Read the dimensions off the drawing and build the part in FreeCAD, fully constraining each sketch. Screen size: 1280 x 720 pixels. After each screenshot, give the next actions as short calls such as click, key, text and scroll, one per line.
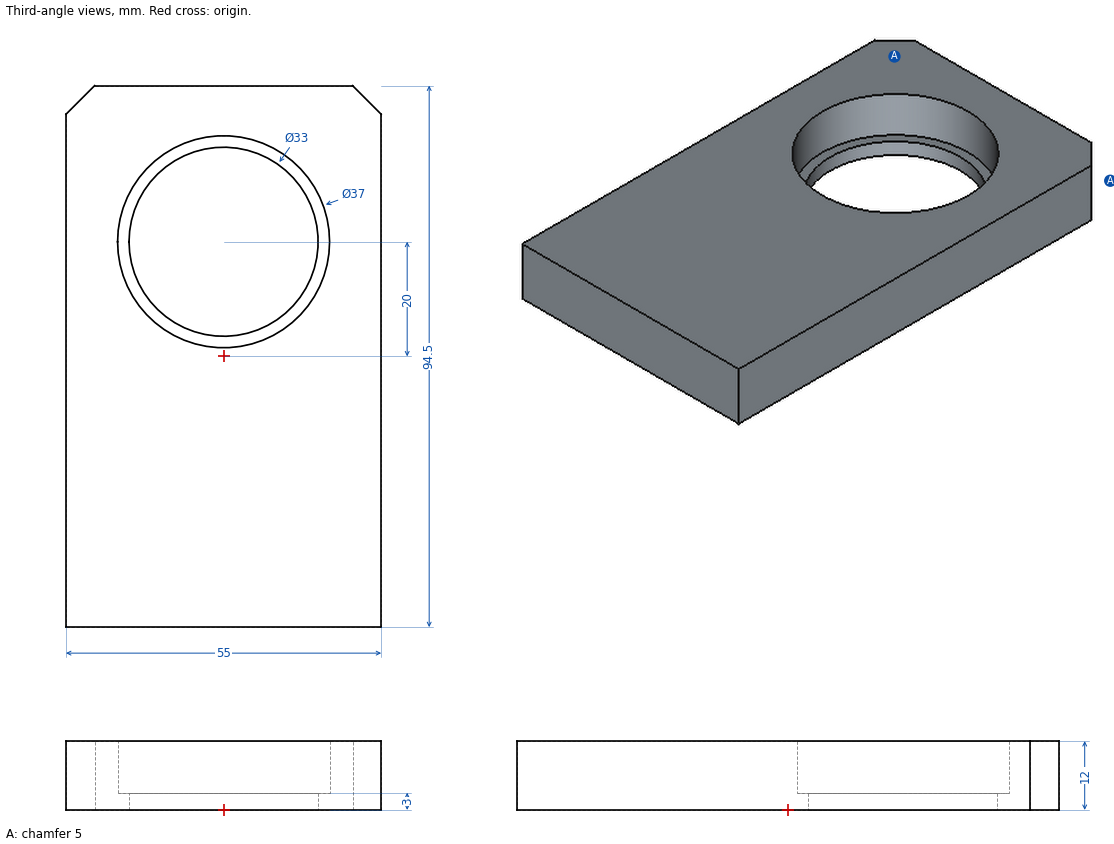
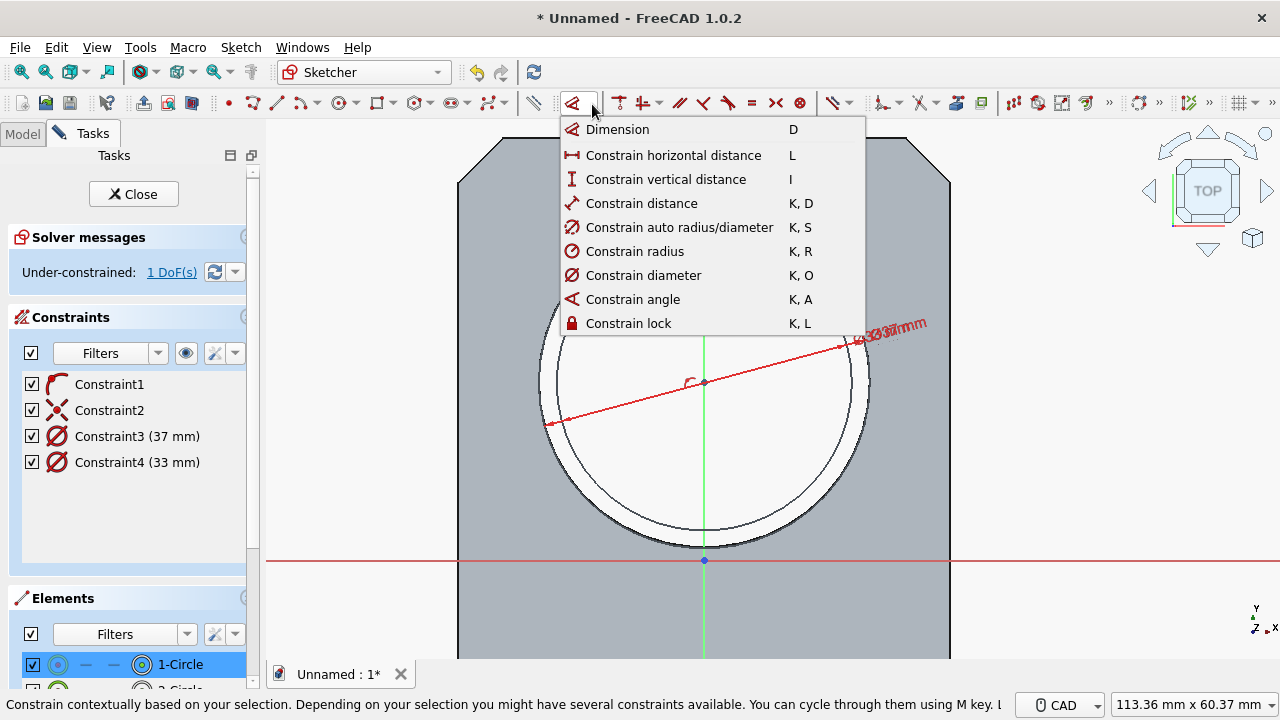
click(713, 179)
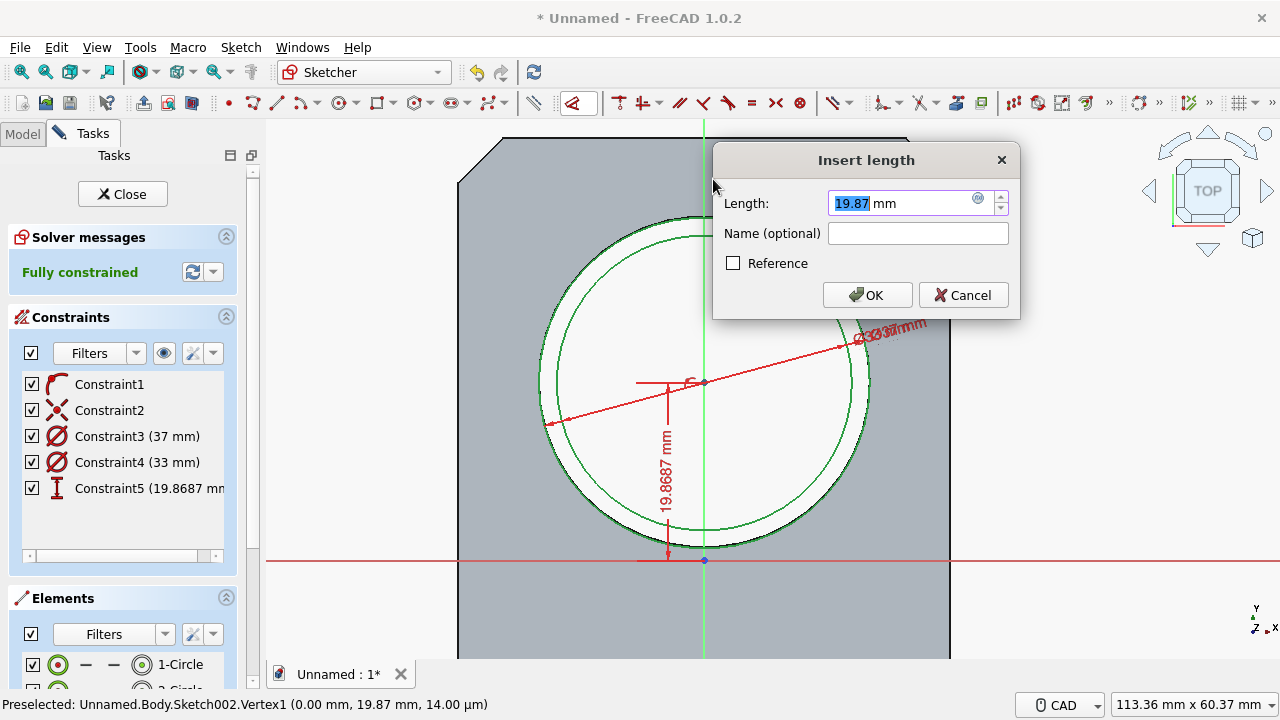
text(20)
key(Return)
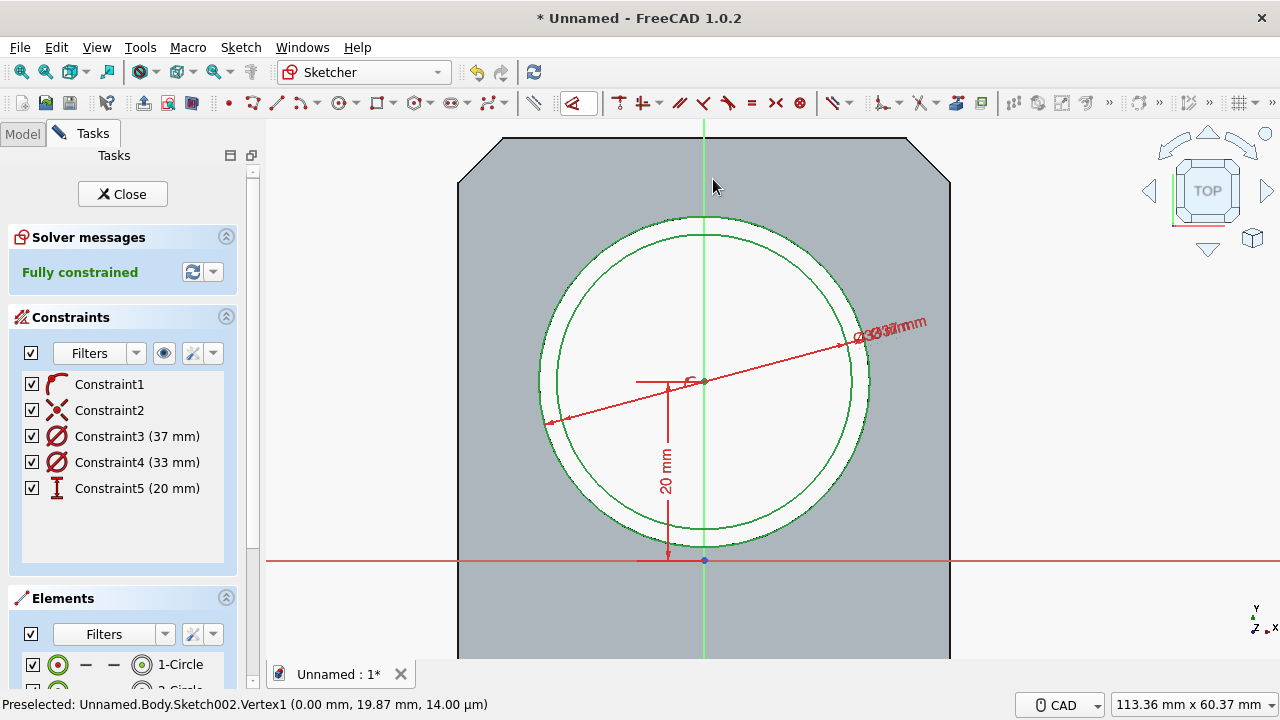
click(123, 194)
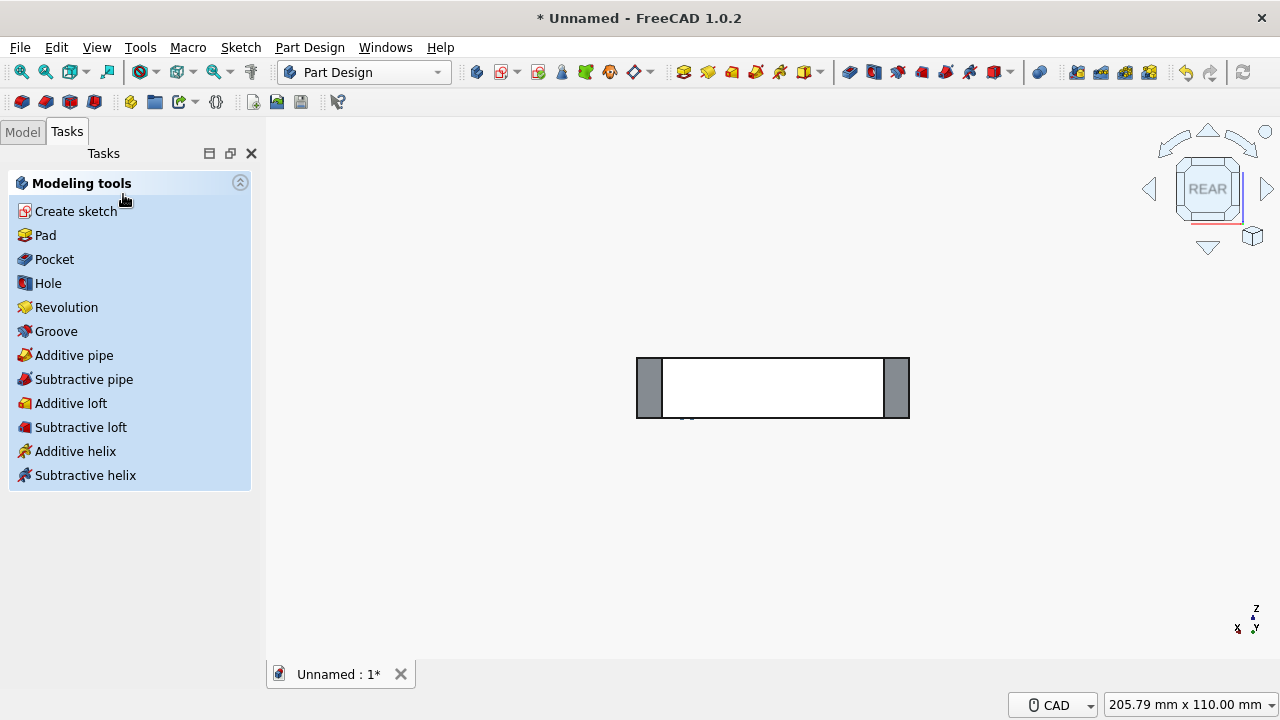
click(684, 72)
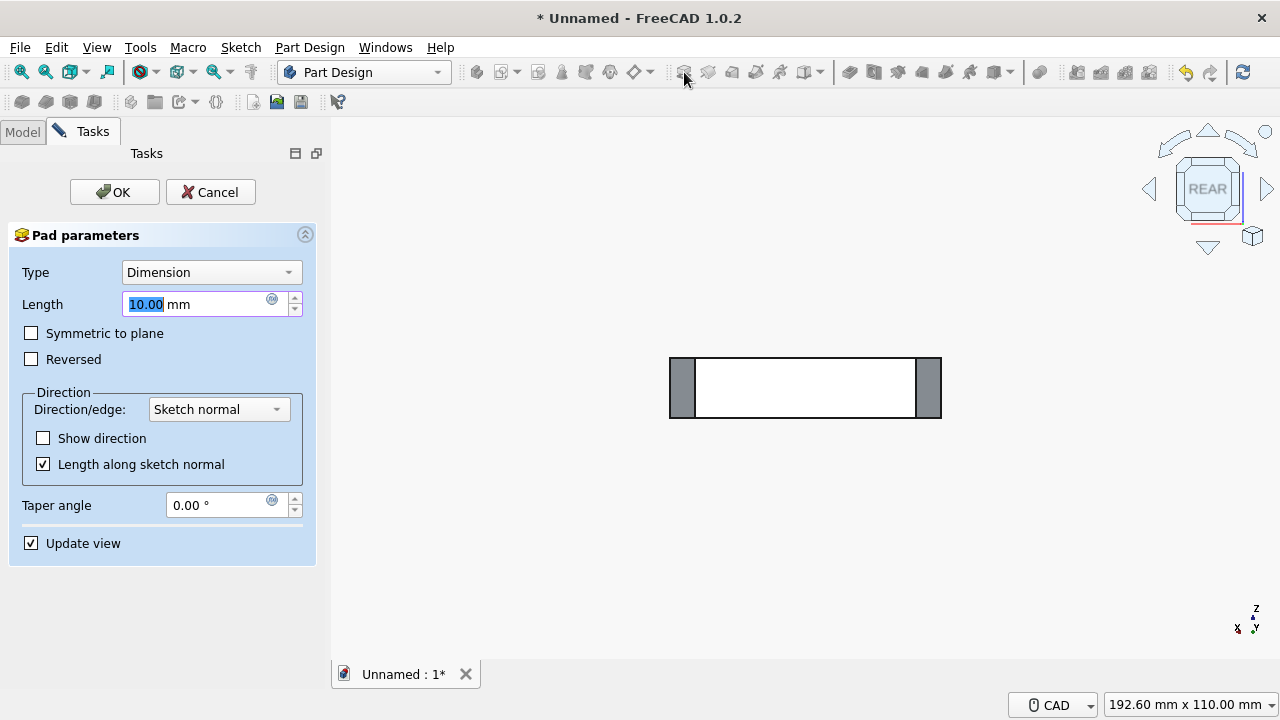
text(3)
key(Tab)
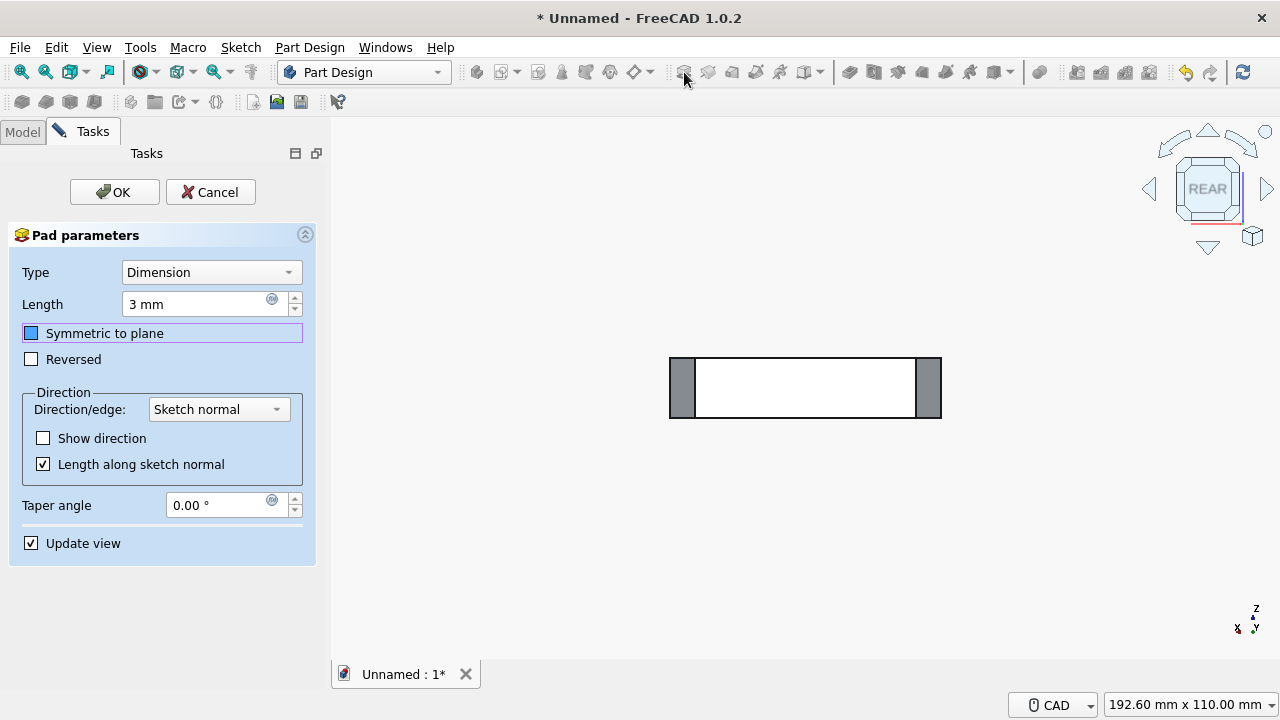
click(115, 192)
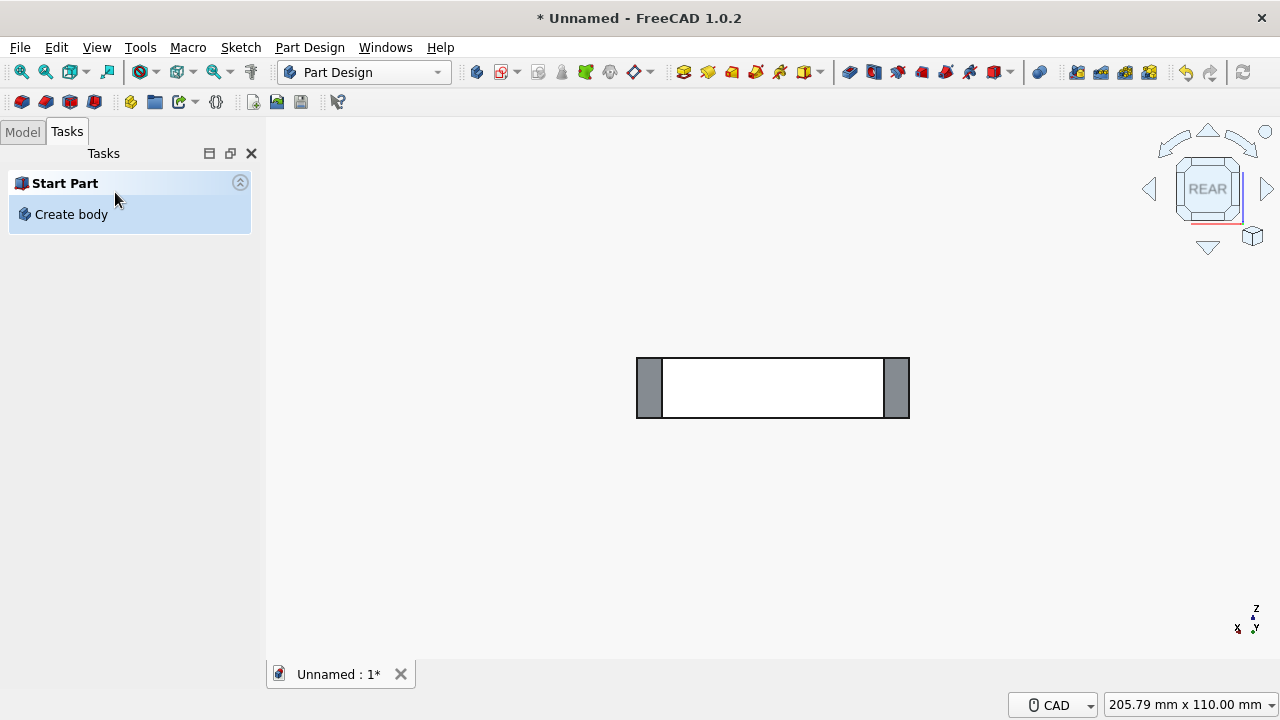
key(0)